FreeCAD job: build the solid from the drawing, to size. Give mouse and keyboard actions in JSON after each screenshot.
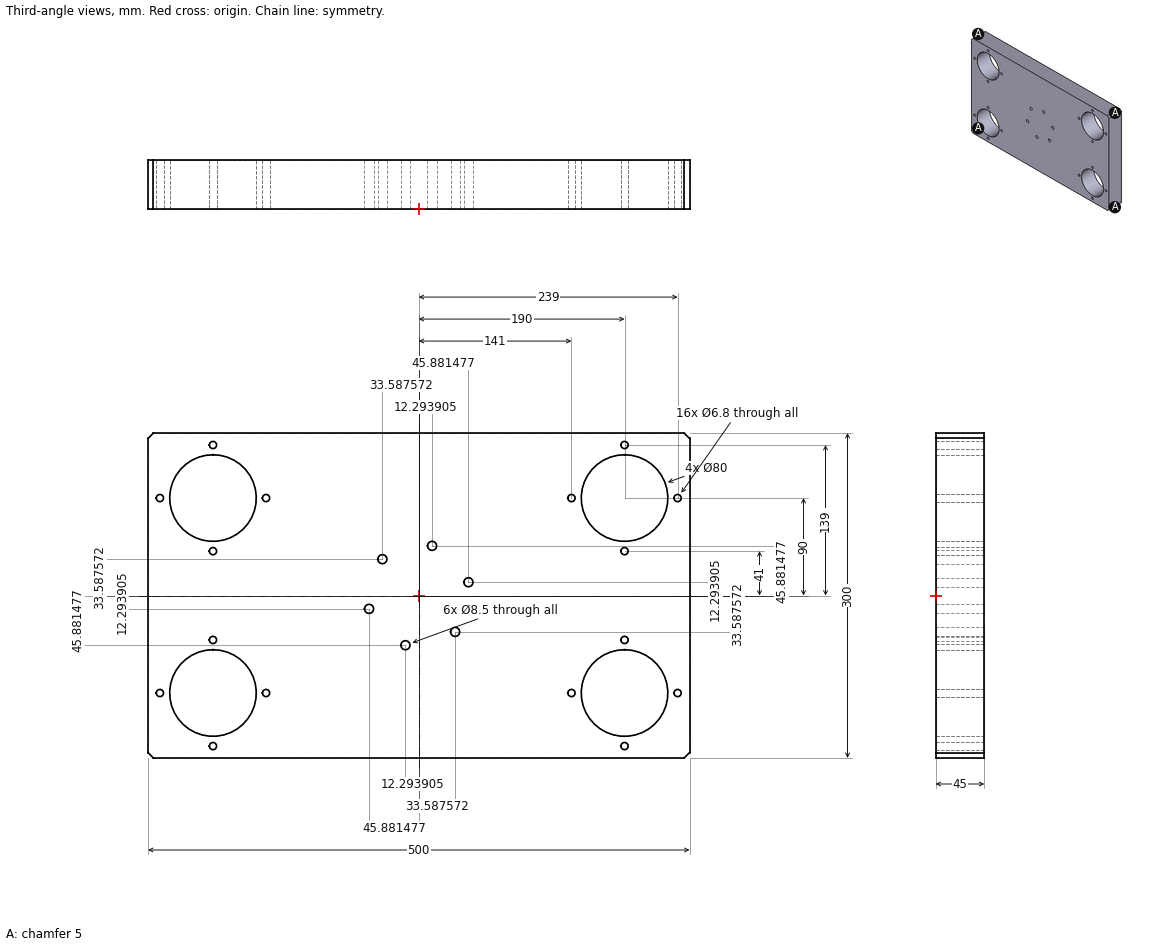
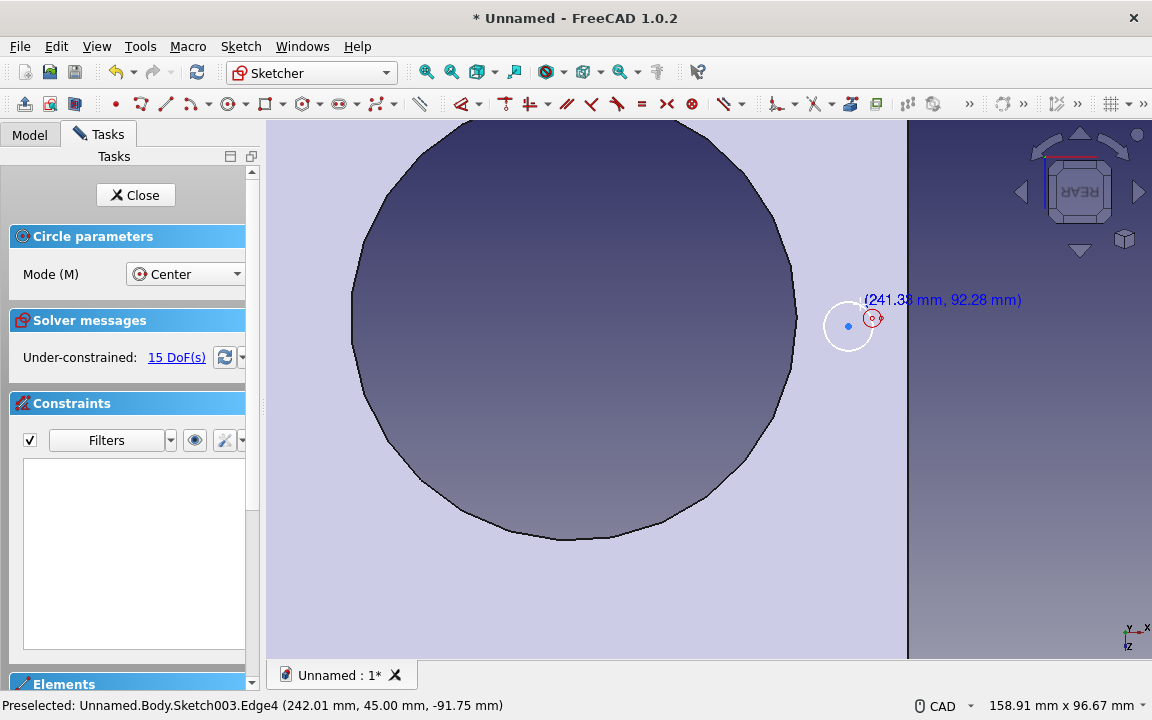
{"action": "scroll", "coordinate": [864, 304], "scroll_direction": "down", "scroll_amount": 9}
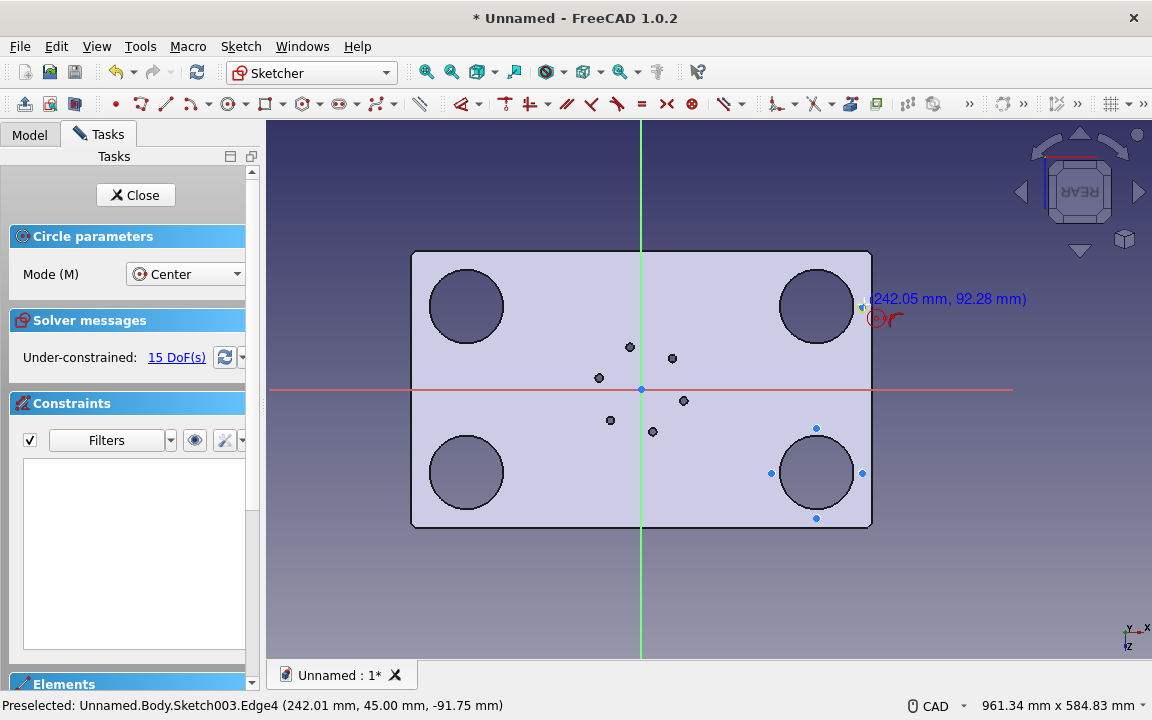
{"action": "left_click", "coordinate": [817, 352]}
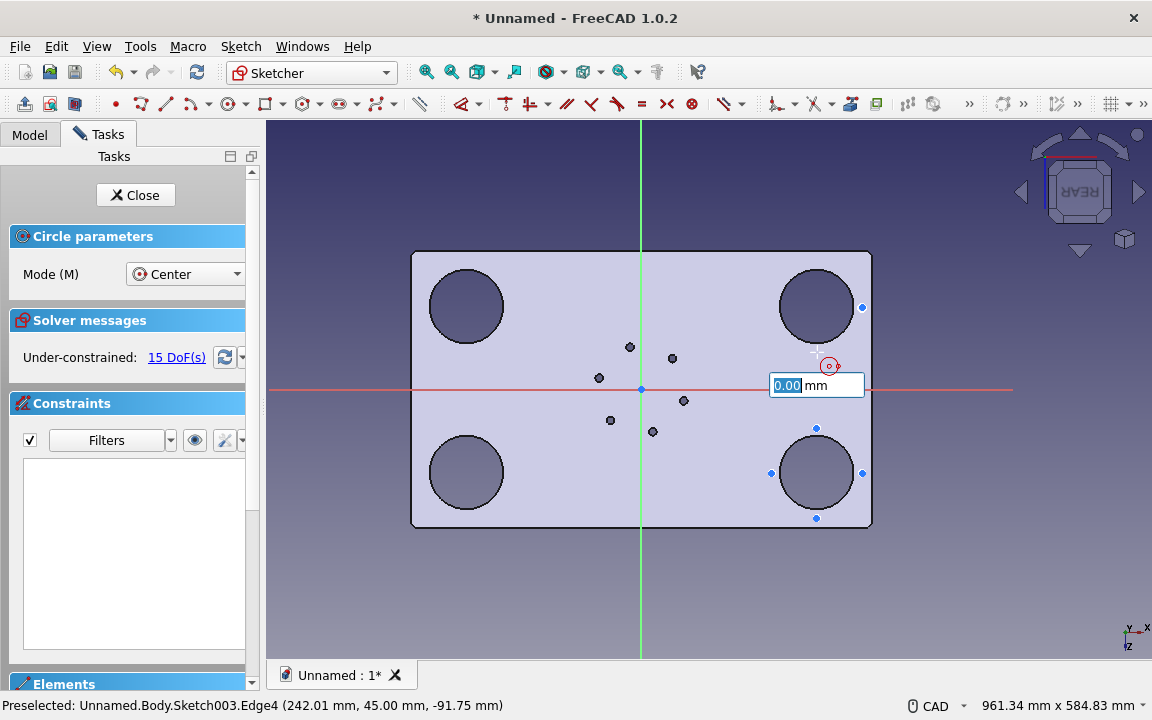
{"action": "scroll", "coordinate": [819, 349], "scroll_direction": "up", "scroll_amount": 9}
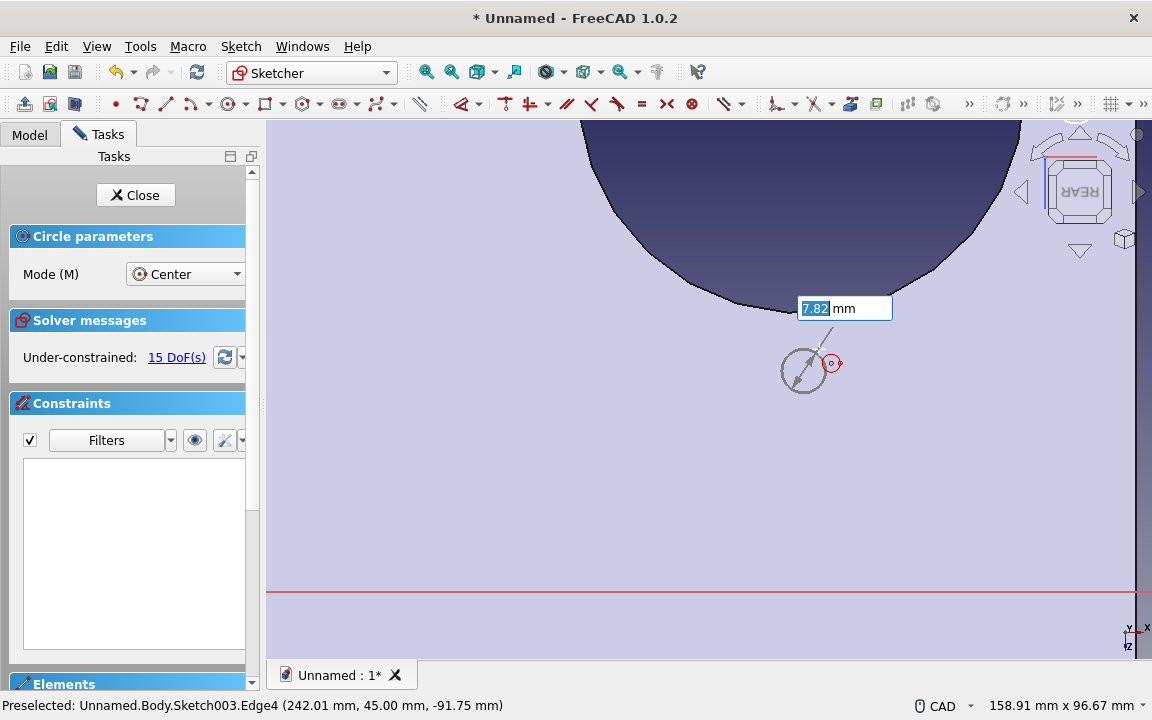
{"action": "left_click", "coordinate": [815, 350]}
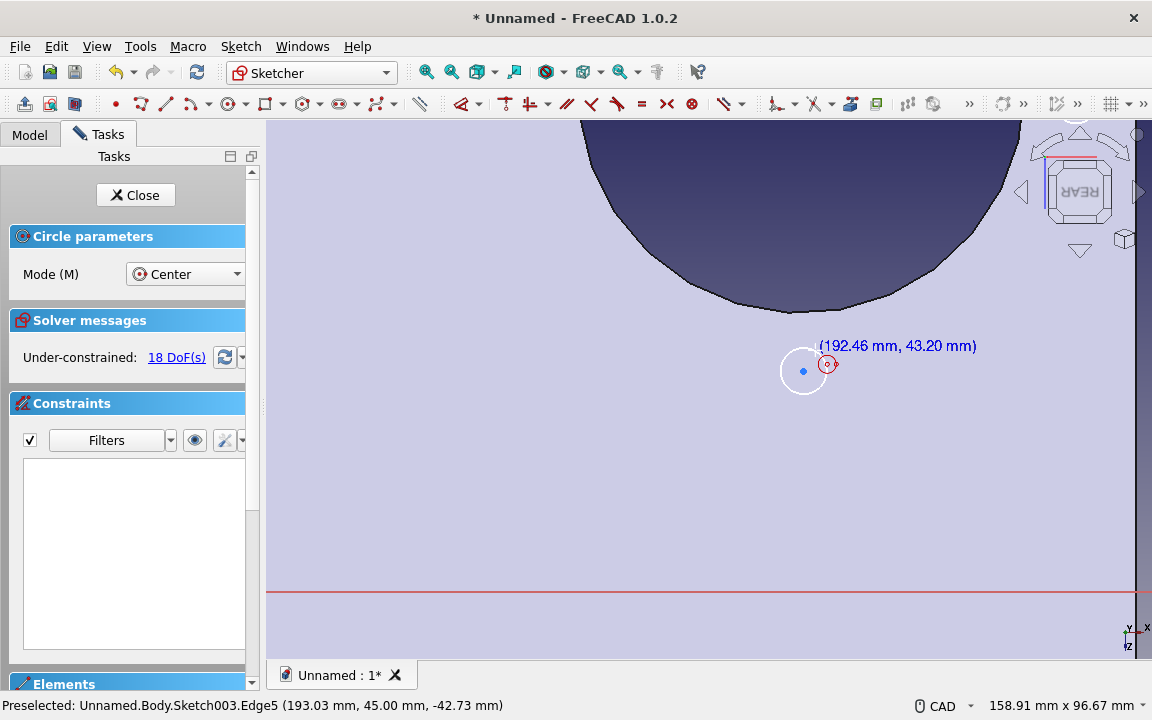
{"action": "scroll", "coordinate": [818, 349], "scroll_direction": "down", "scroll_amount": 9}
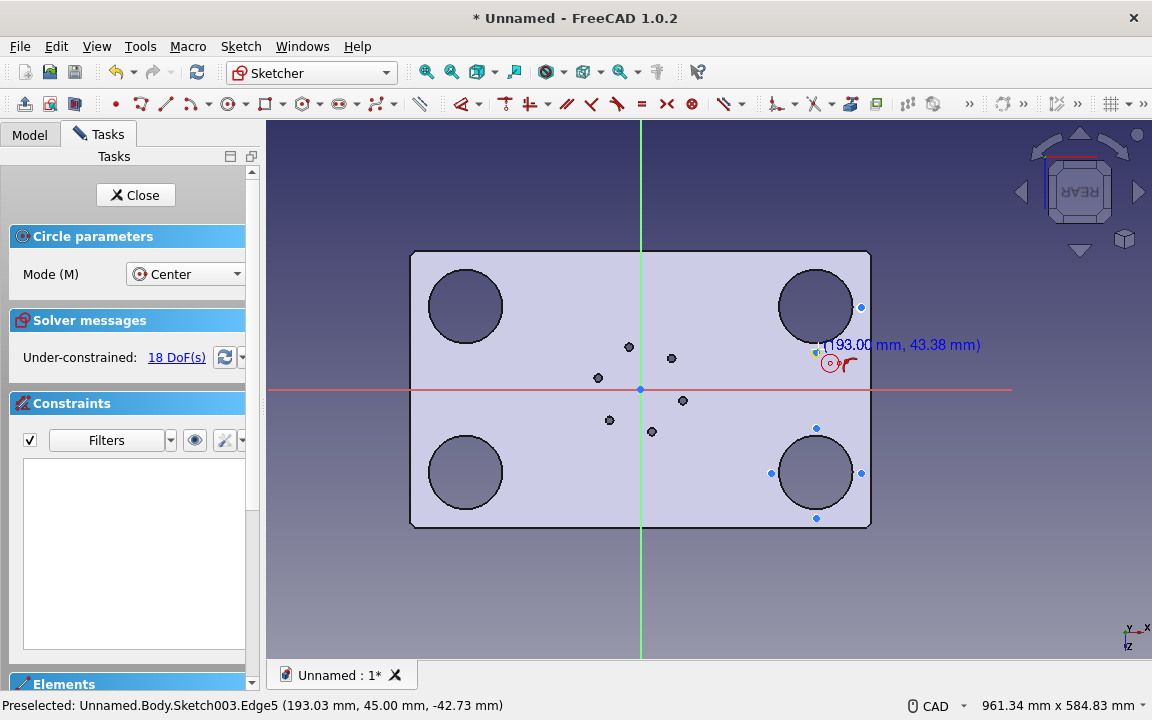
{"action": "scroll", "coordinate": [771, 307], "scroll_direction": "up", "scroll_amount": 10}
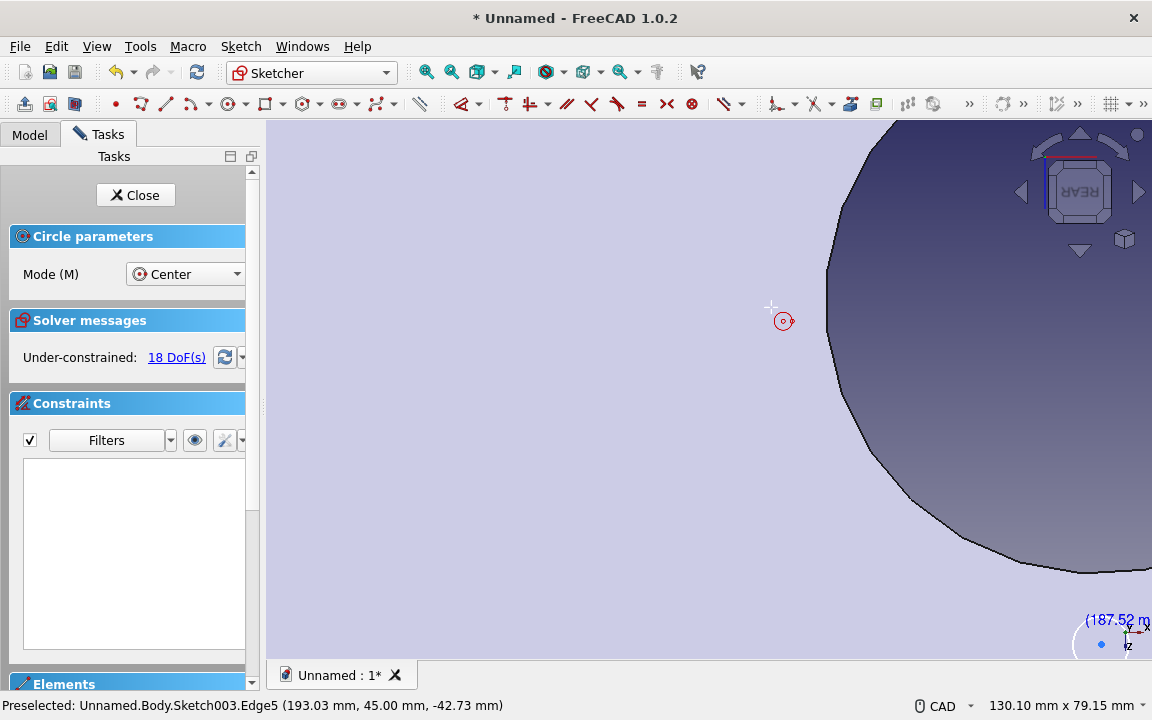
{"action": "scroll", "coordinate": [771, 307], "scroll_direction": "down", "scroll_amount": 10}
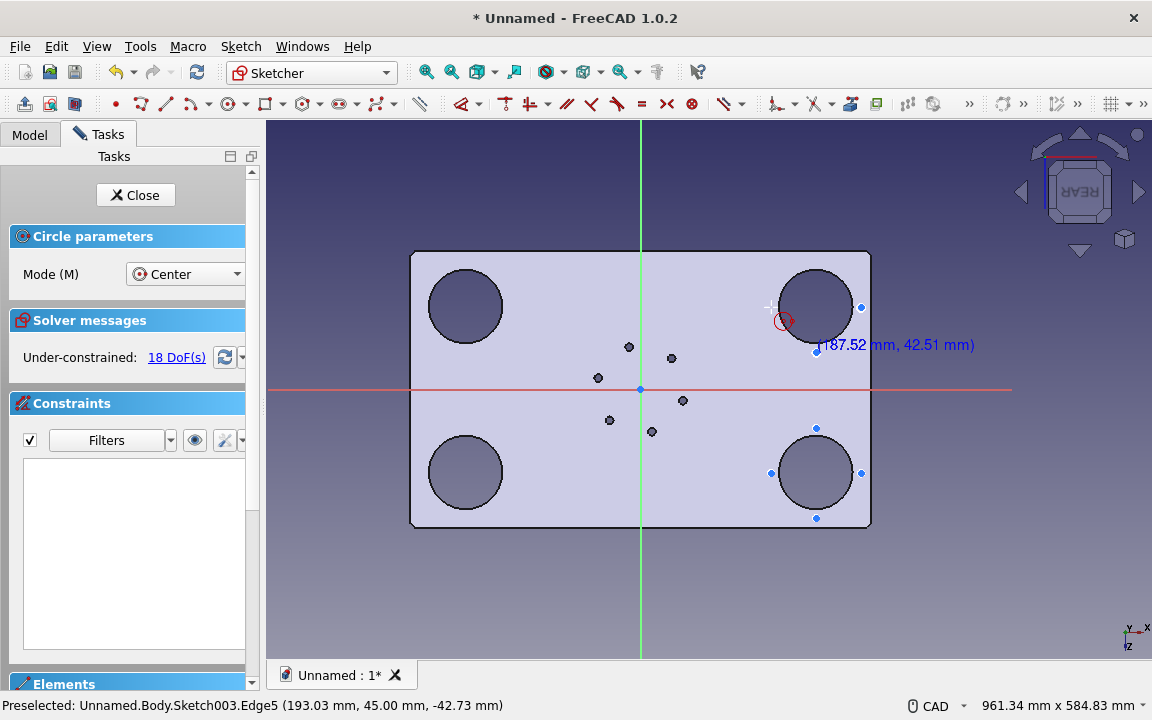
{"action": "left_click", "coordinate": [771, 307]}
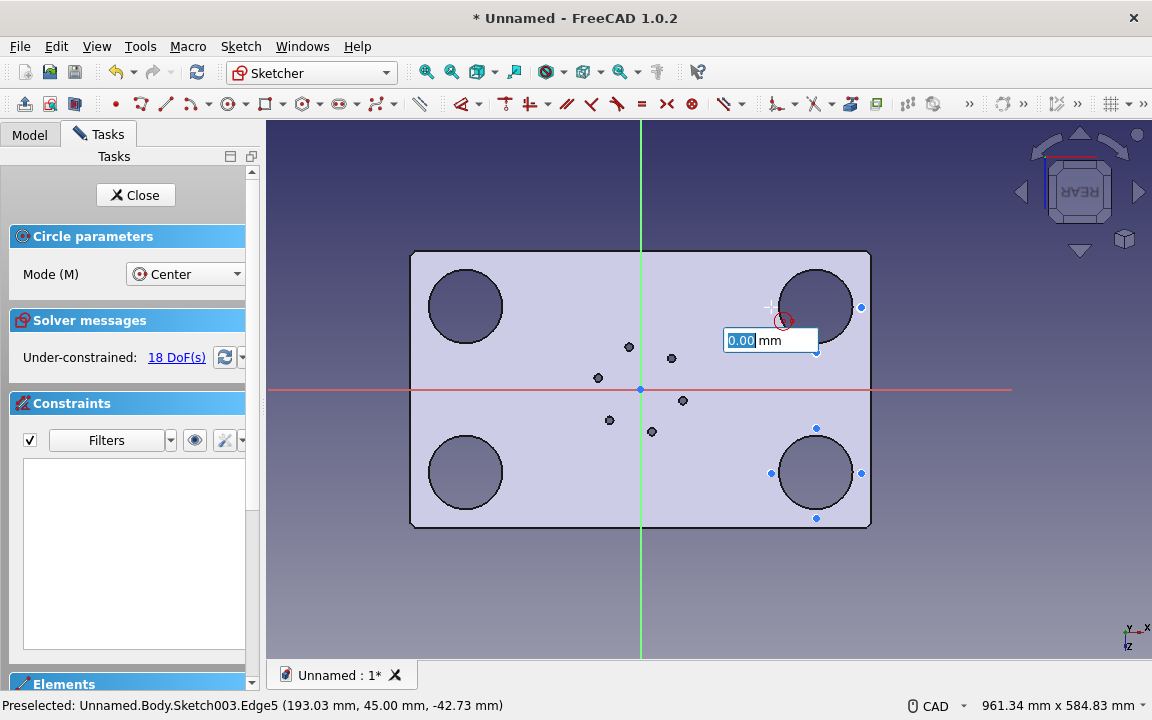
{"action": "scroll", "coordinate": [773, 304], "scroll_direction": "up", "scroll_amount": 9}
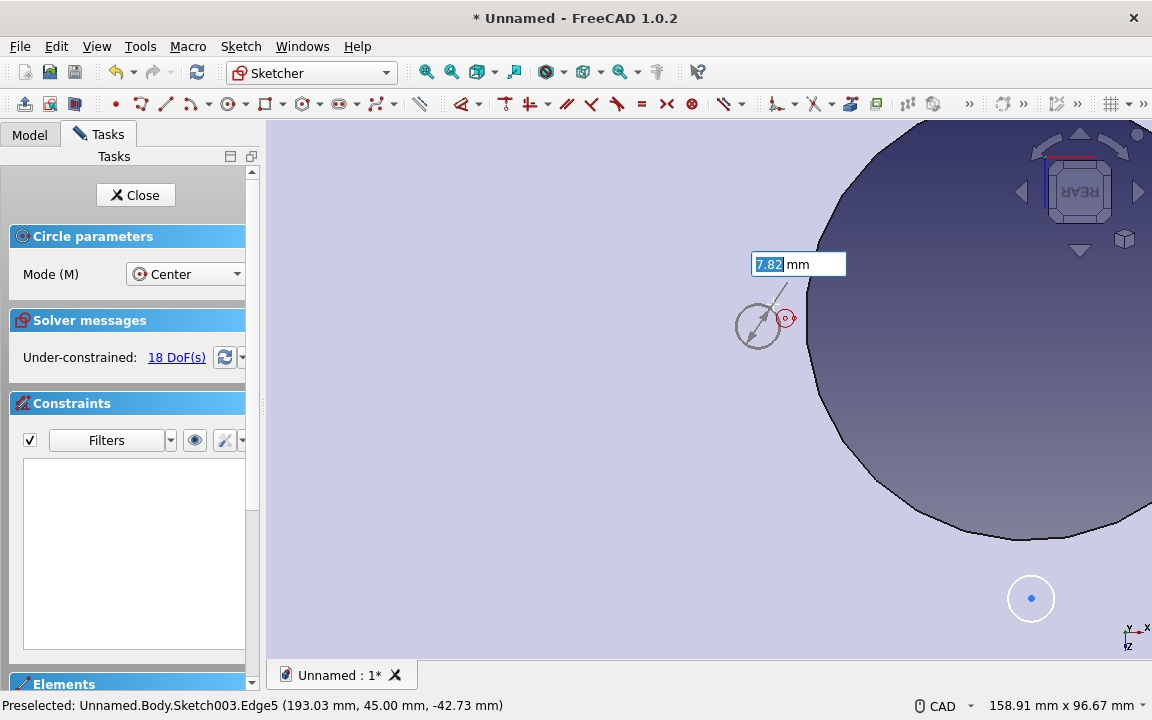
{"action": "left_click", "coordinate": [769, 304]}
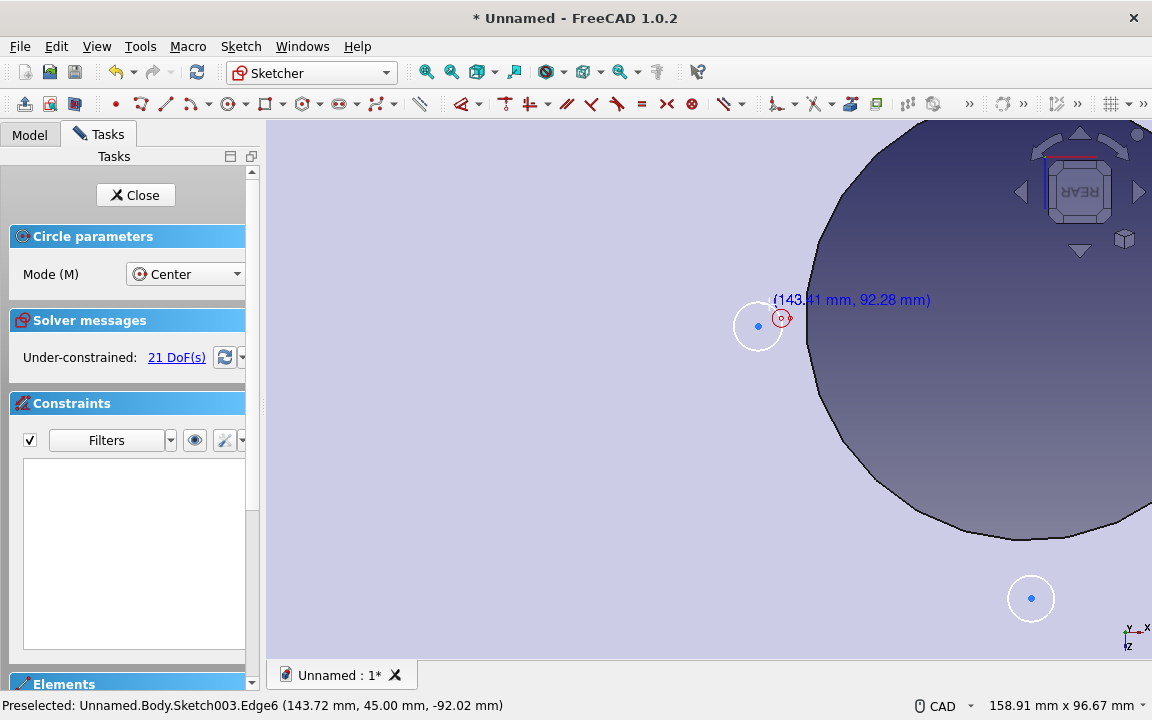
{"action": "scroll", "coordinate": [773, 304], "scroll_direction": "down", "scroll_amount": 9}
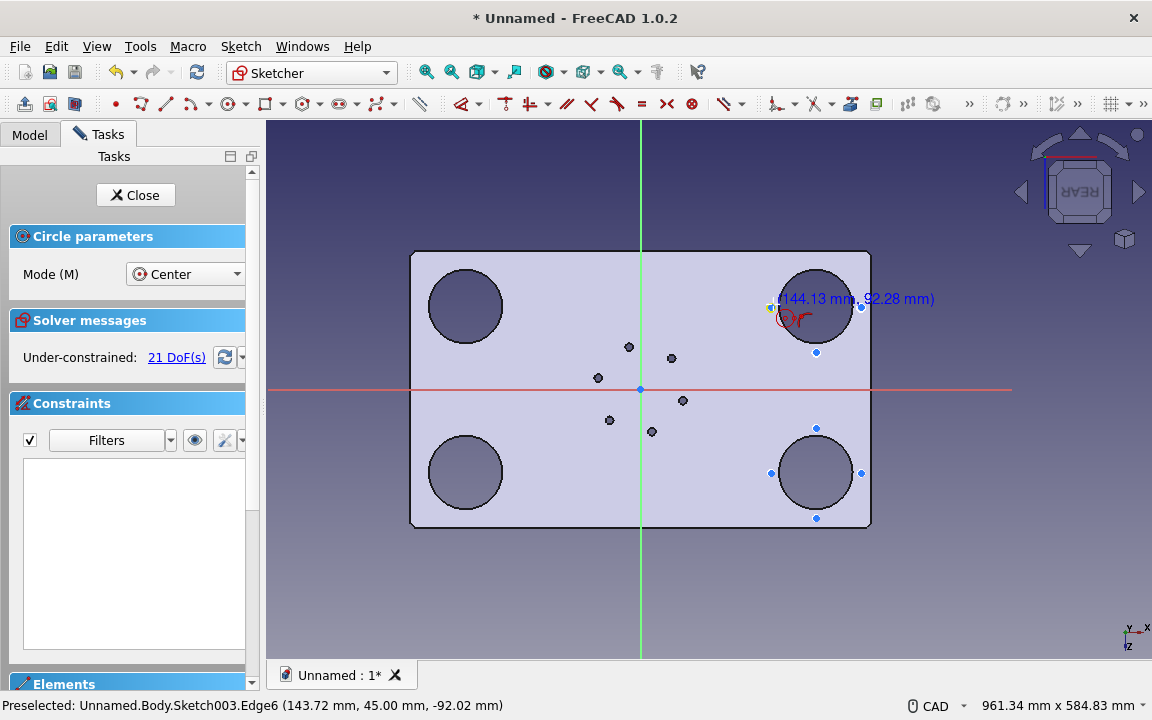
{"action": "scroll", "coordinate": [816, 261], "scroll_direction": "up", "scroll_amount": 10}